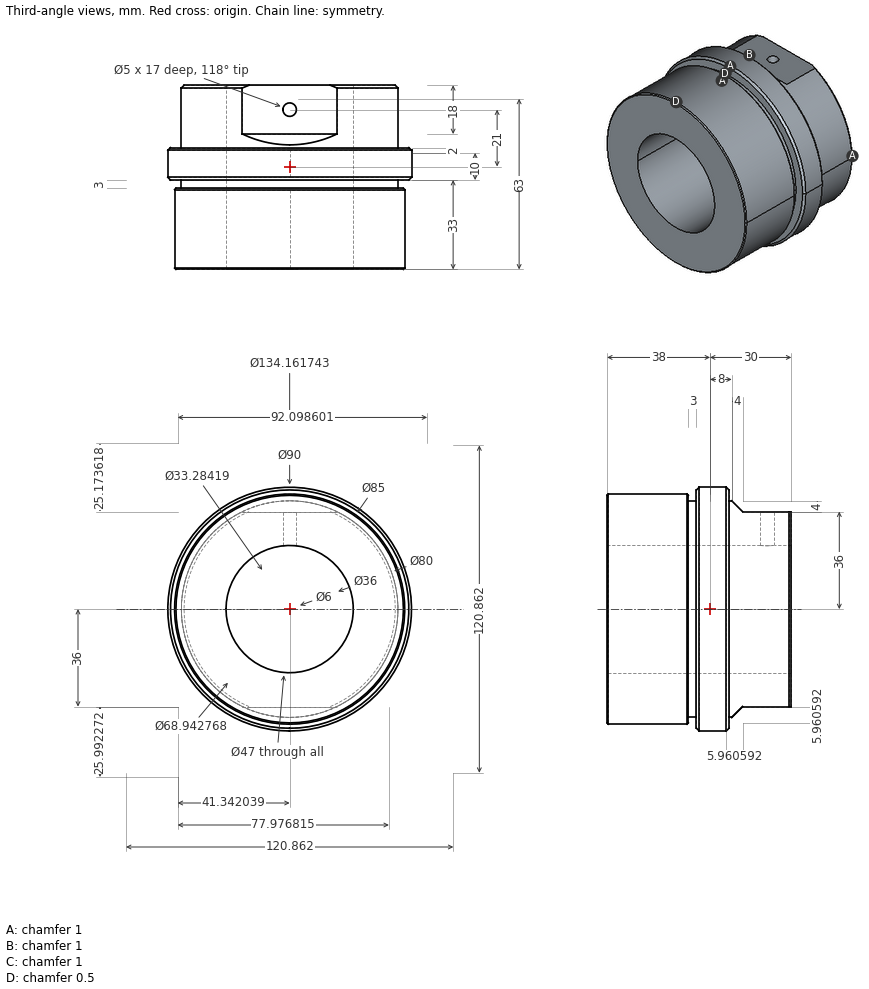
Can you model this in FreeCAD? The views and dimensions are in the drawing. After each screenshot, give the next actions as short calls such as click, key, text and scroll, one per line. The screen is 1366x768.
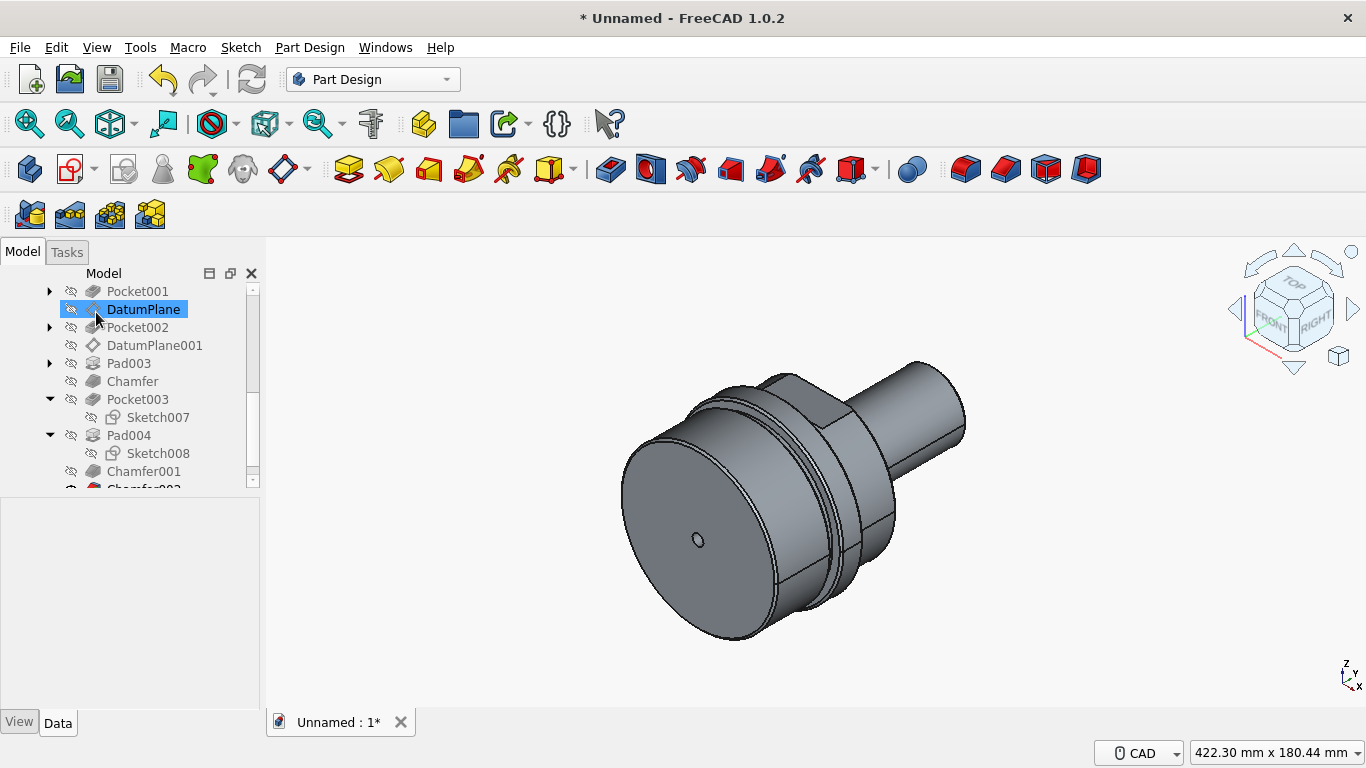
key(5)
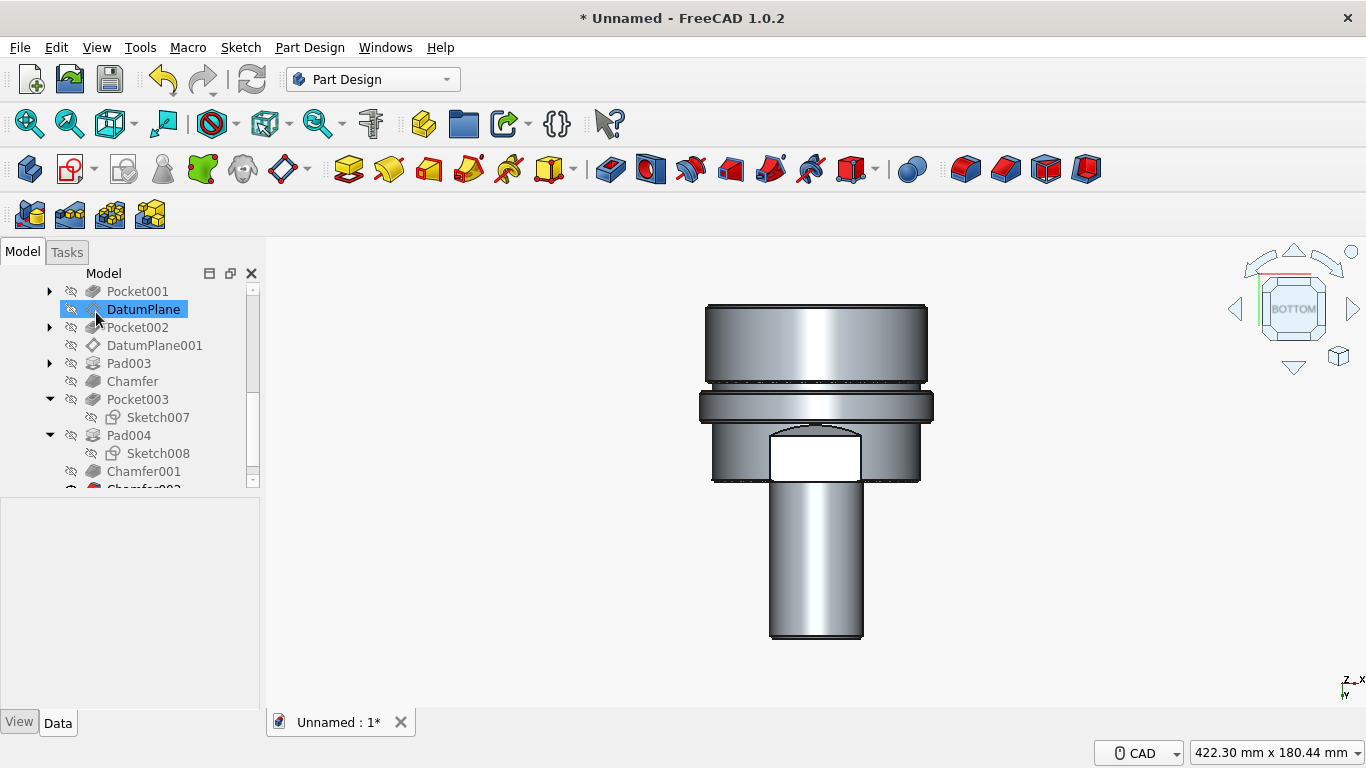
scroll(140, 377, down, 3)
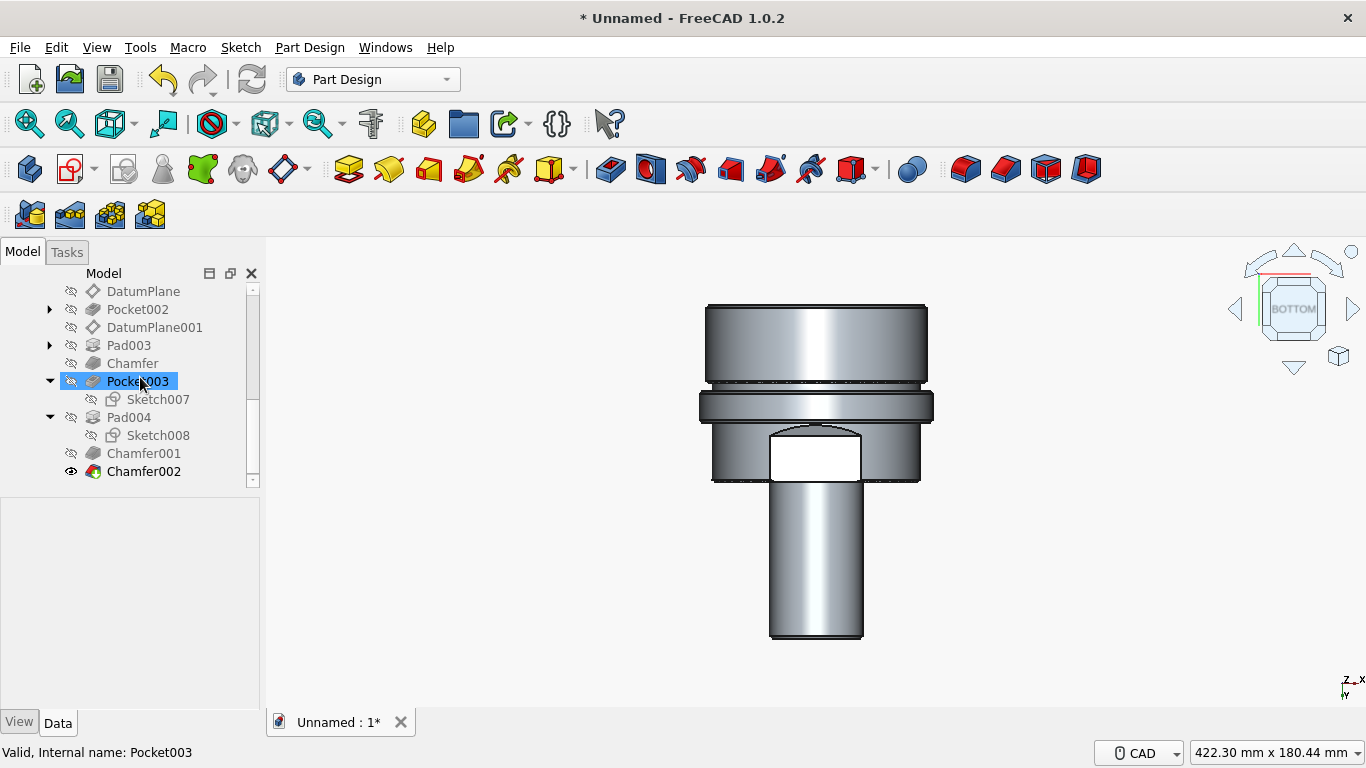
scroll(140, 377, up, 15)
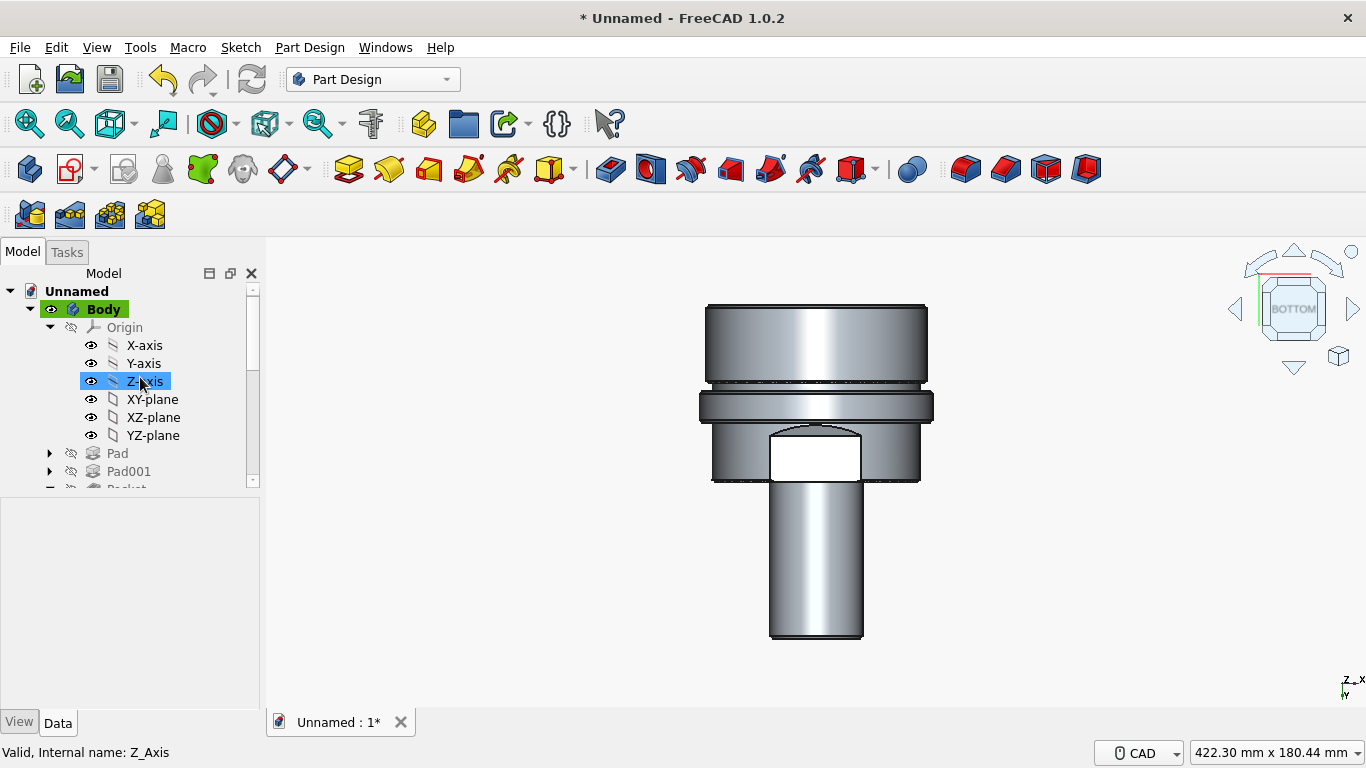
click(136, 417)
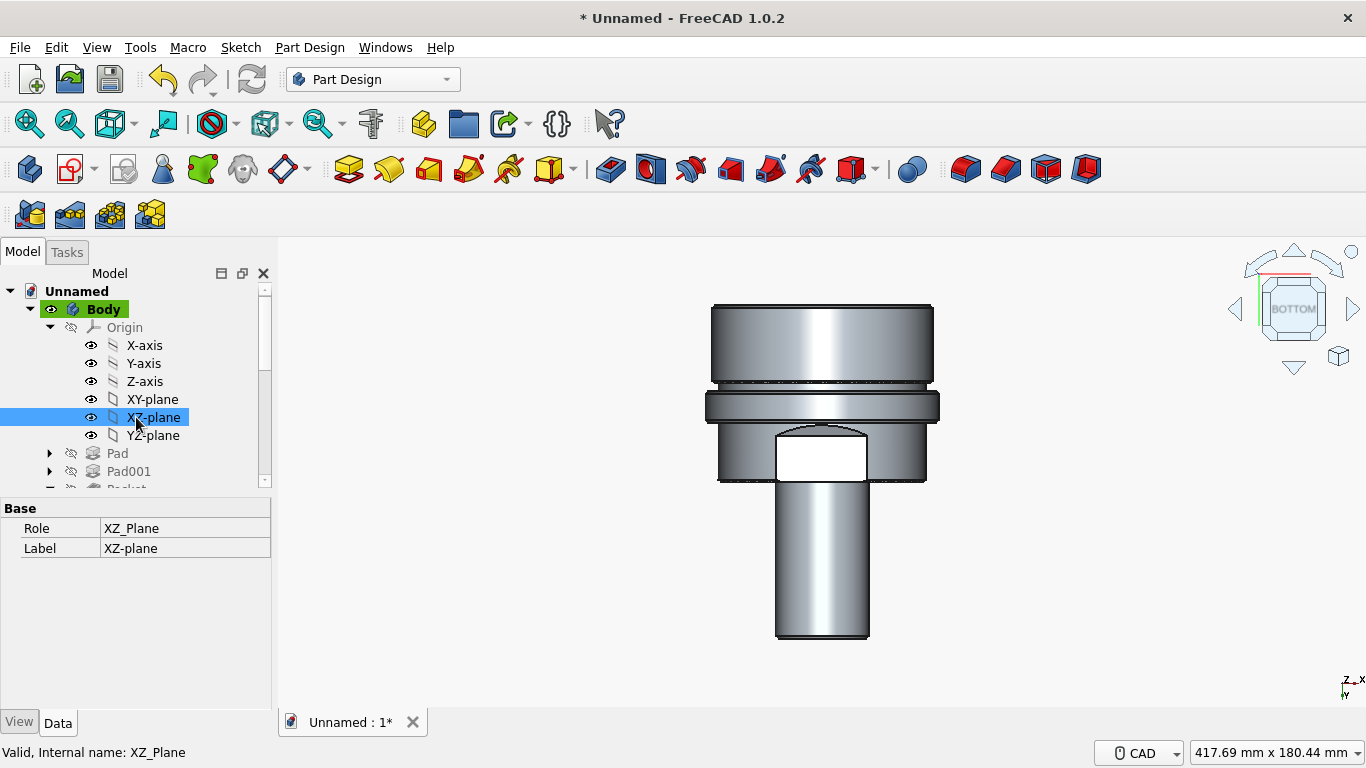
click(284, 170)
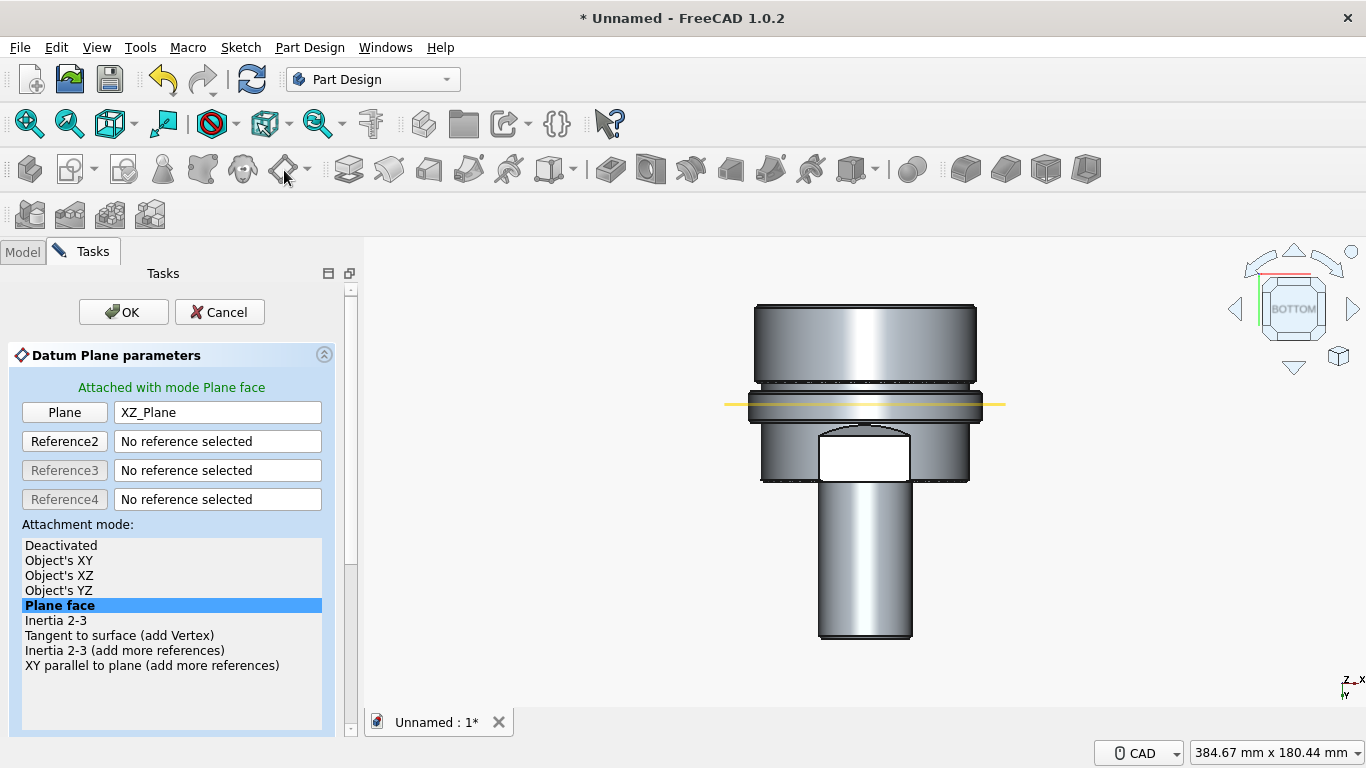
scroll(351, 510, down, 3)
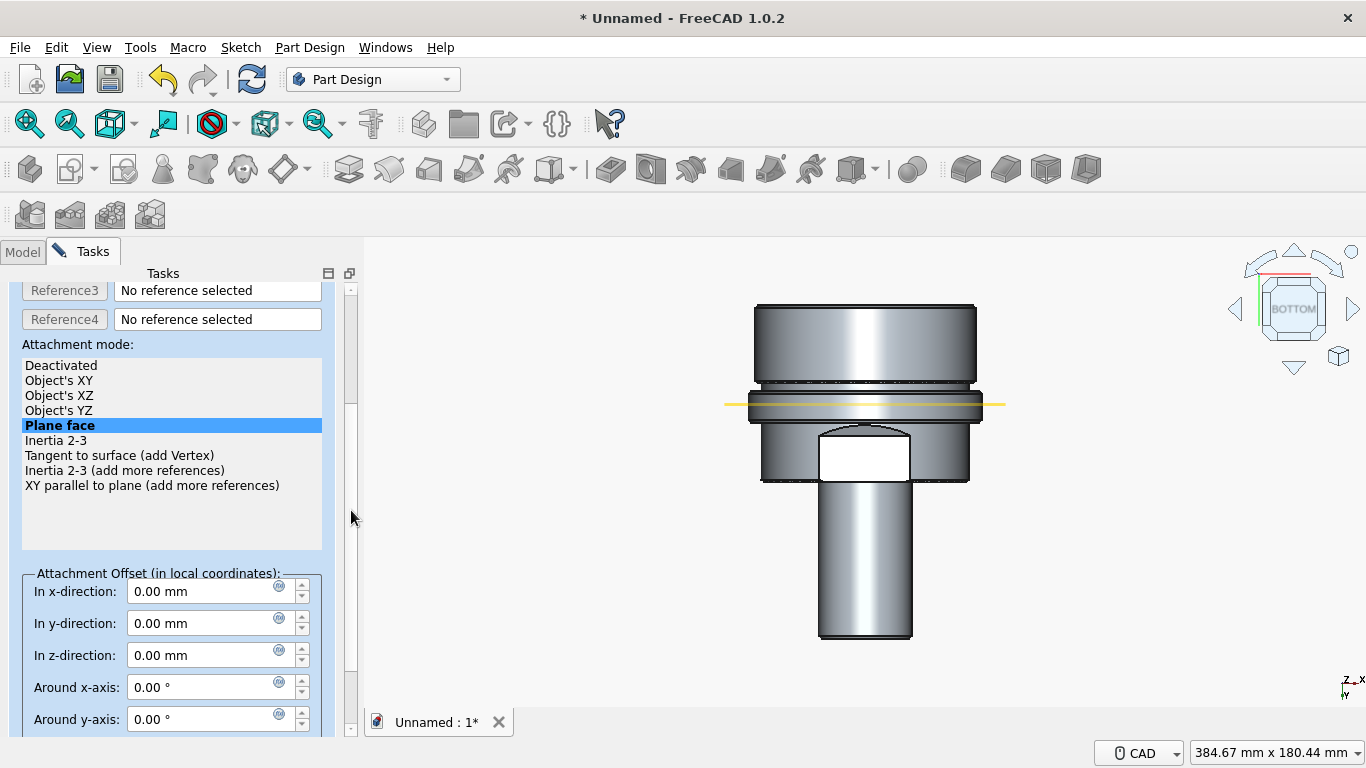
triple_click(210, 655)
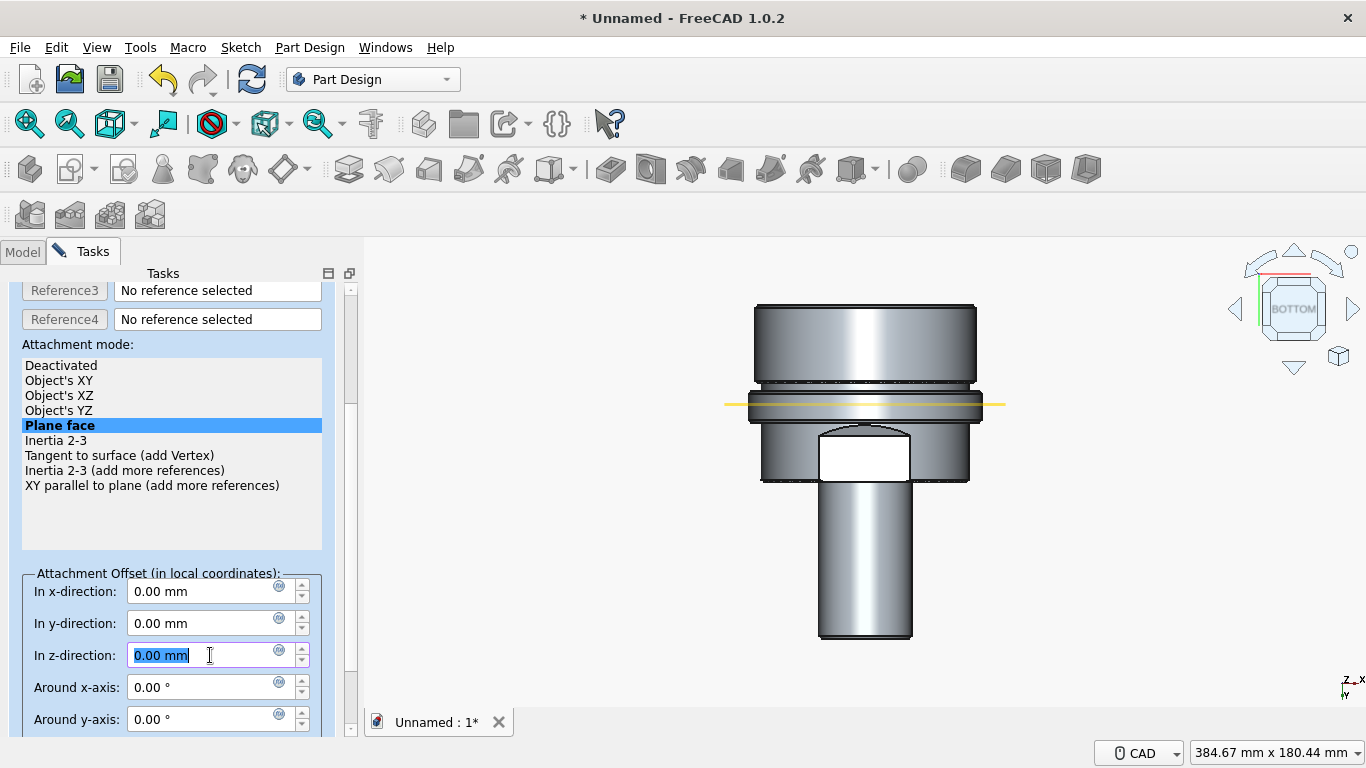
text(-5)
key(Tab)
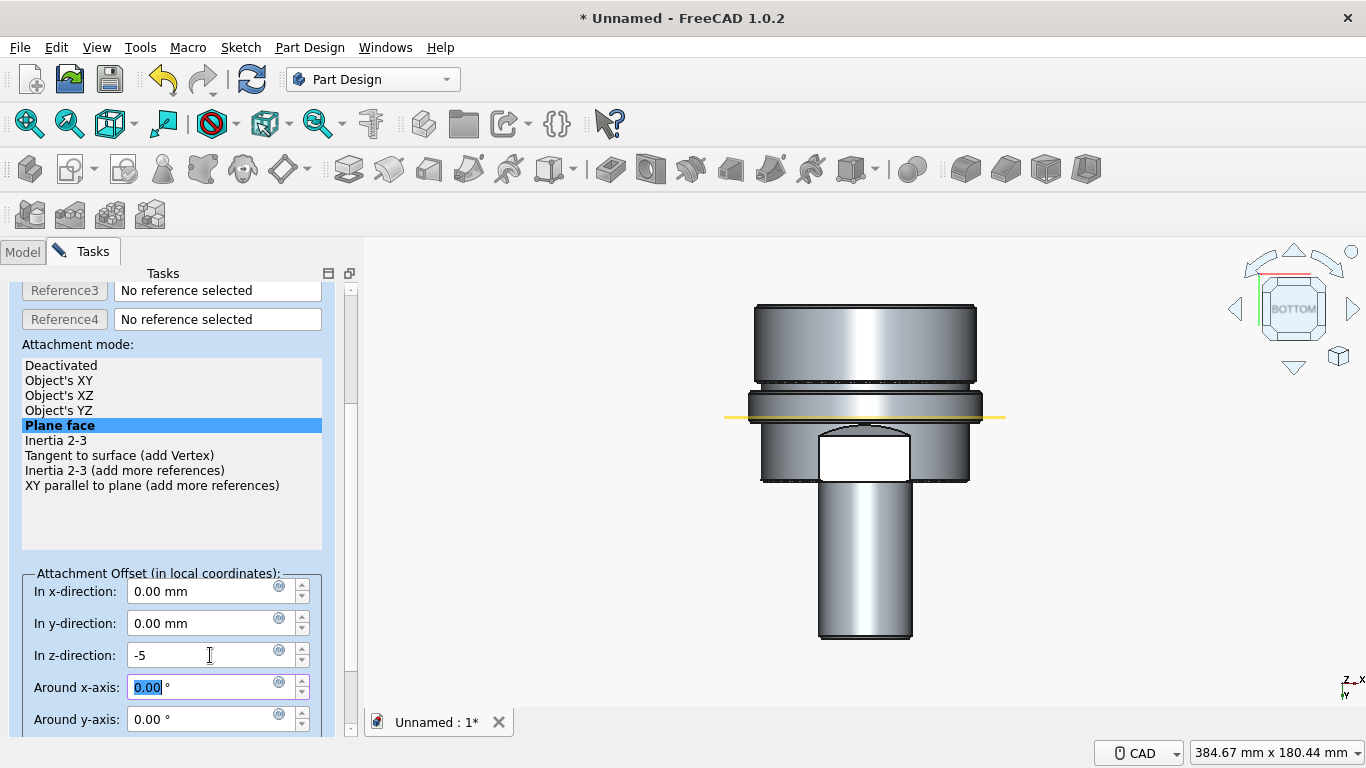
scroll(351, 510, up, 4)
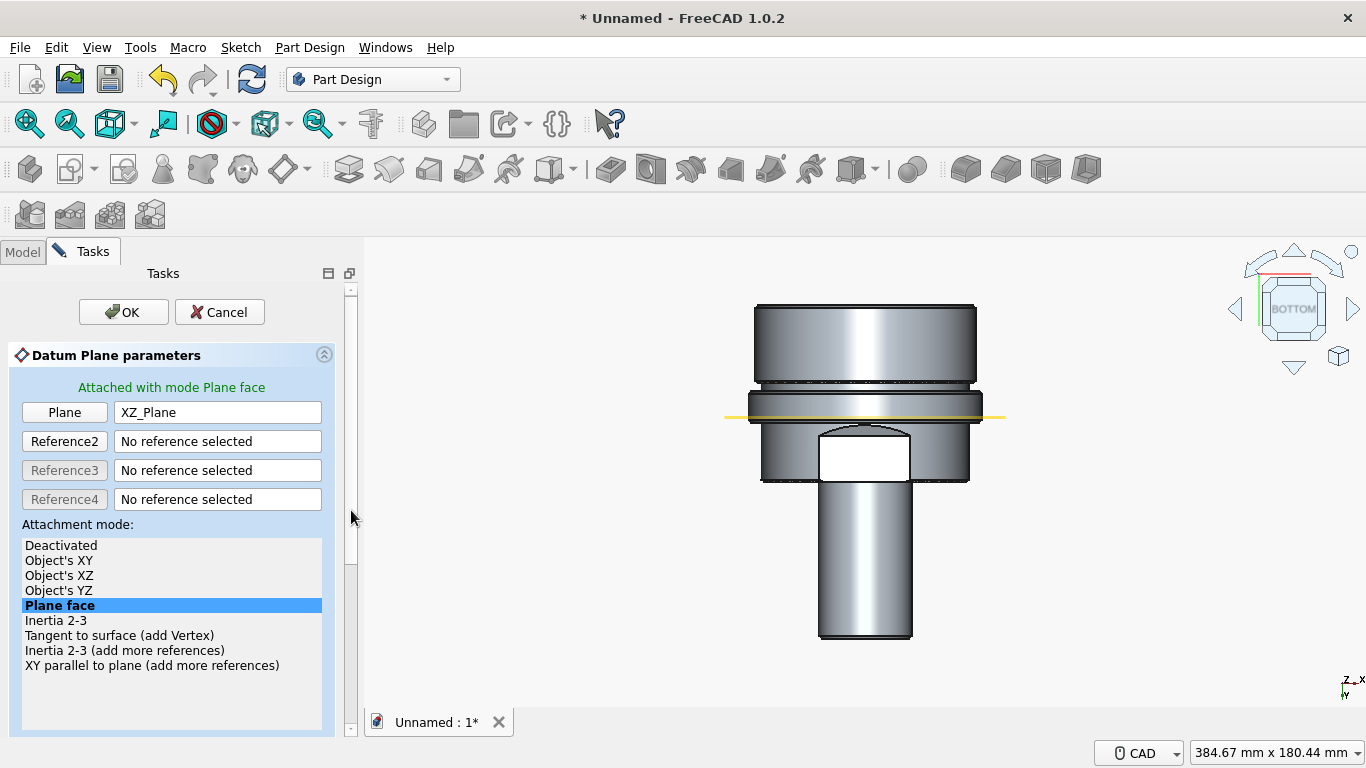
click(124, 312)